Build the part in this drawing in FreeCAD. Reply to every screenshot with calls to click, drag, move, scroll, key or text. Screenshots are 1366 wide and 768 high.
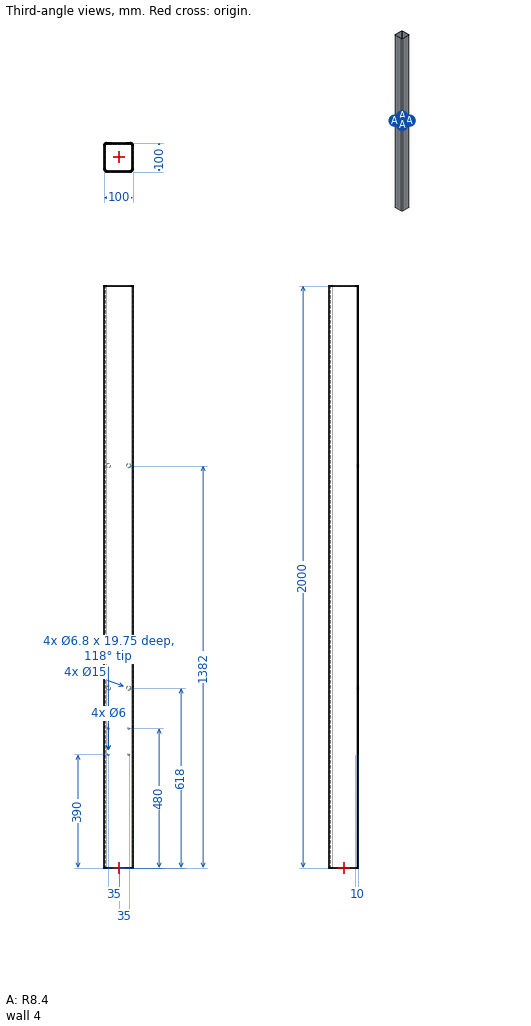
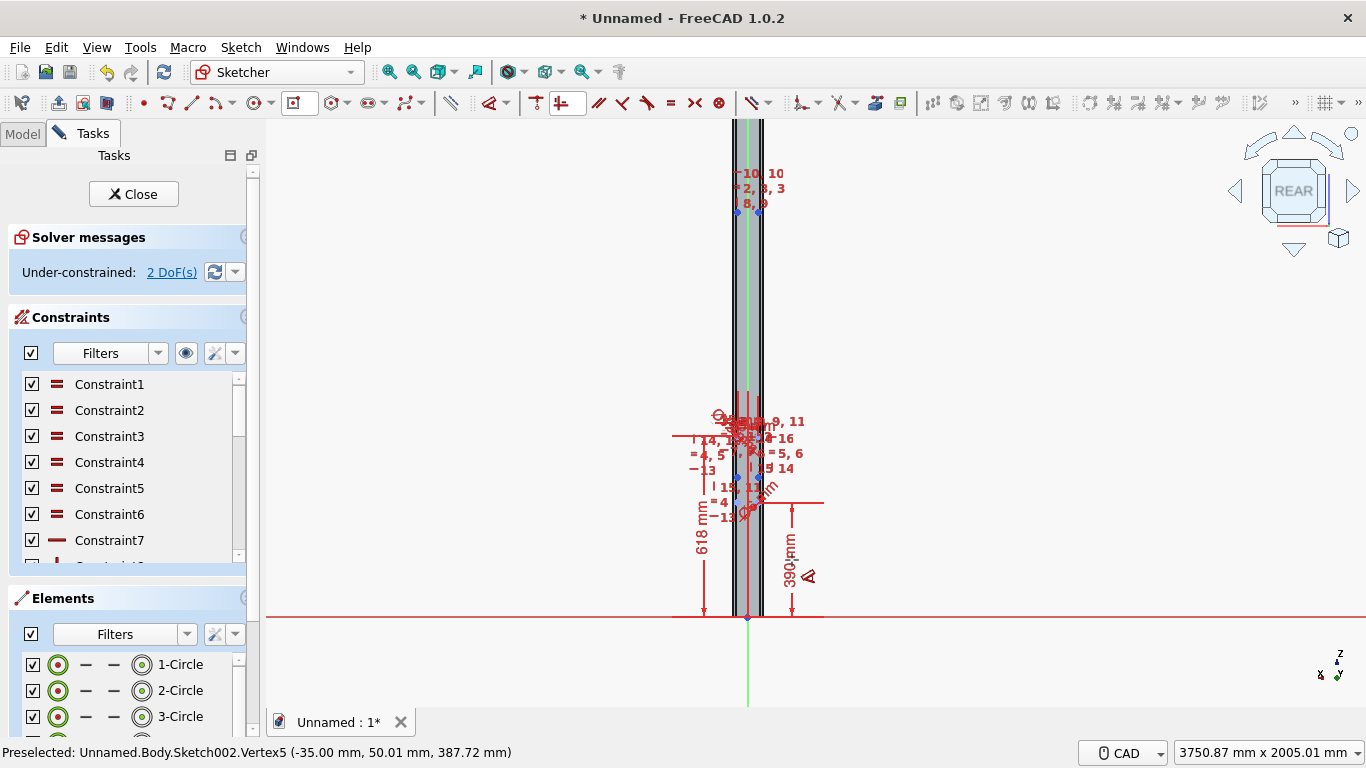
click(738, 477)
click(704, 547)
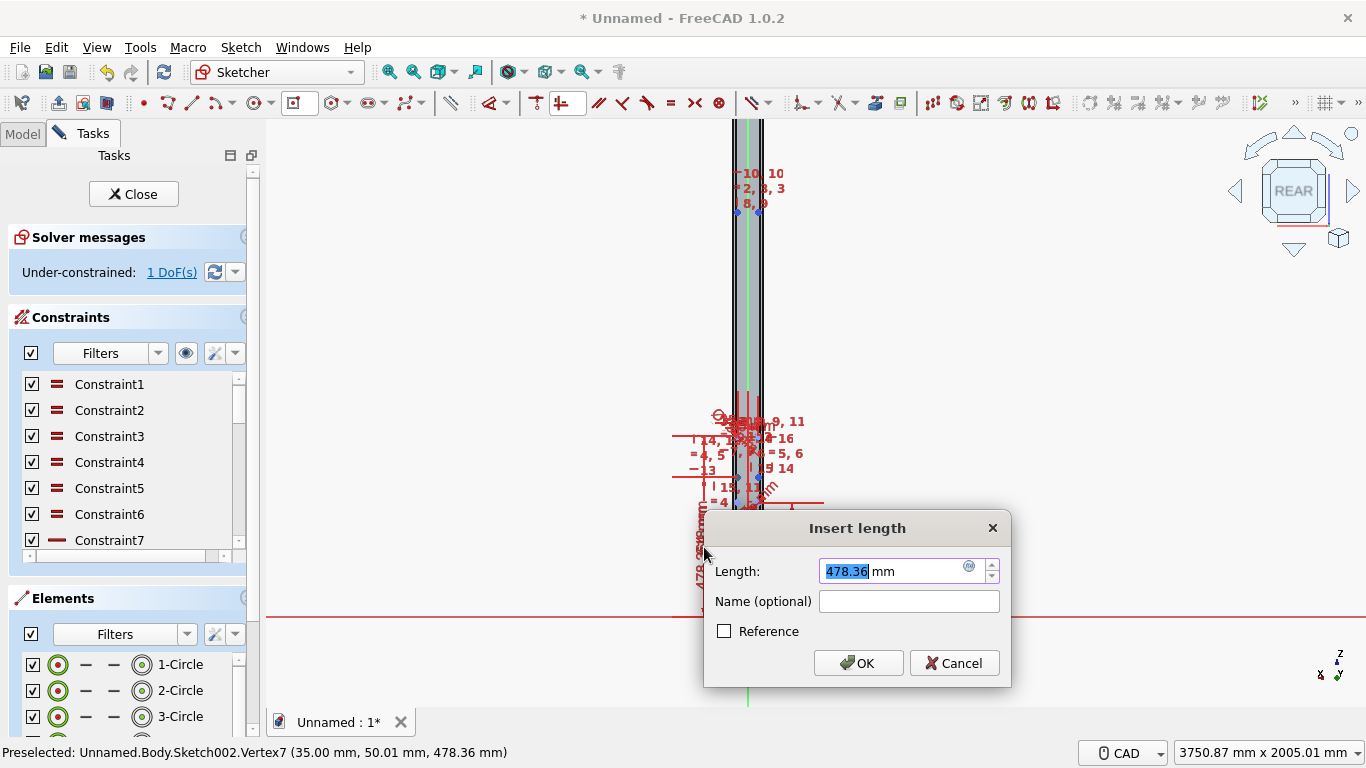
text(480)
key(Return)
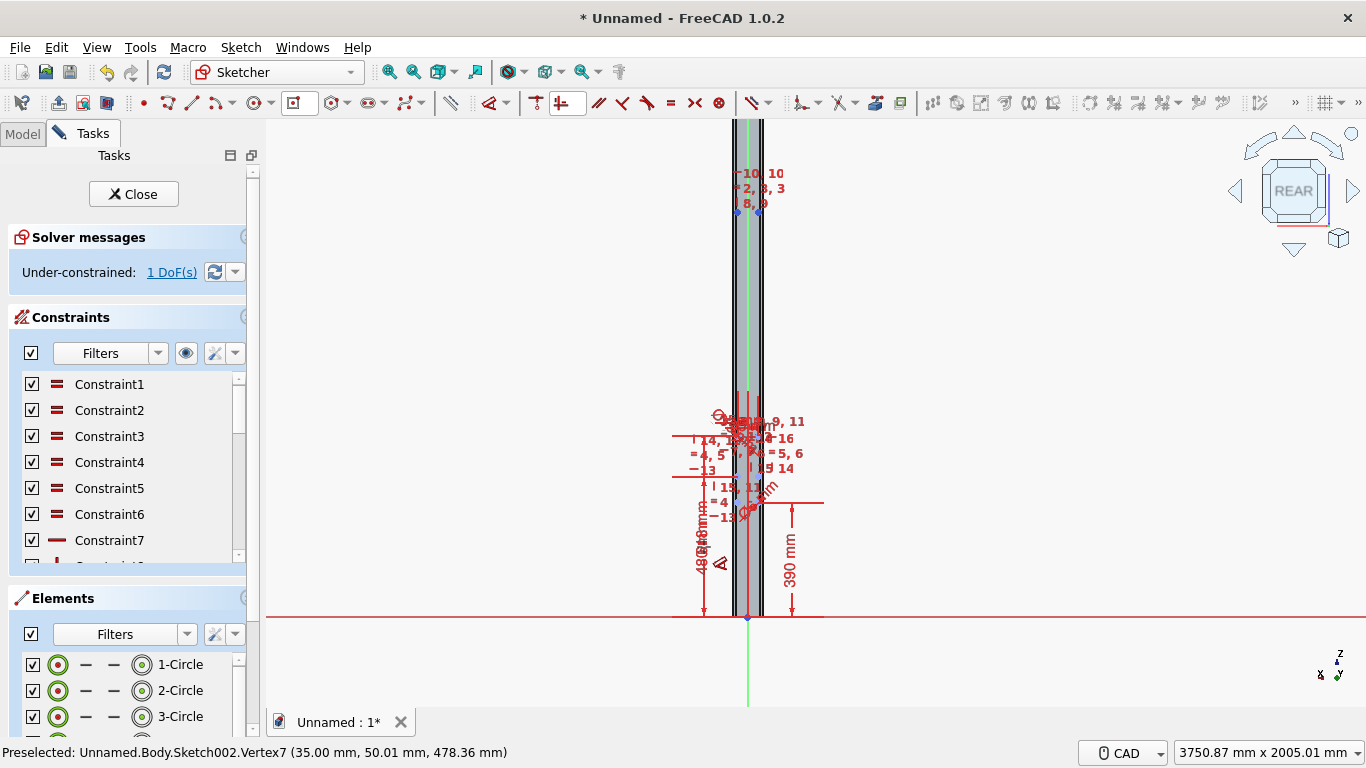
click(738, 212)
click(704, 322)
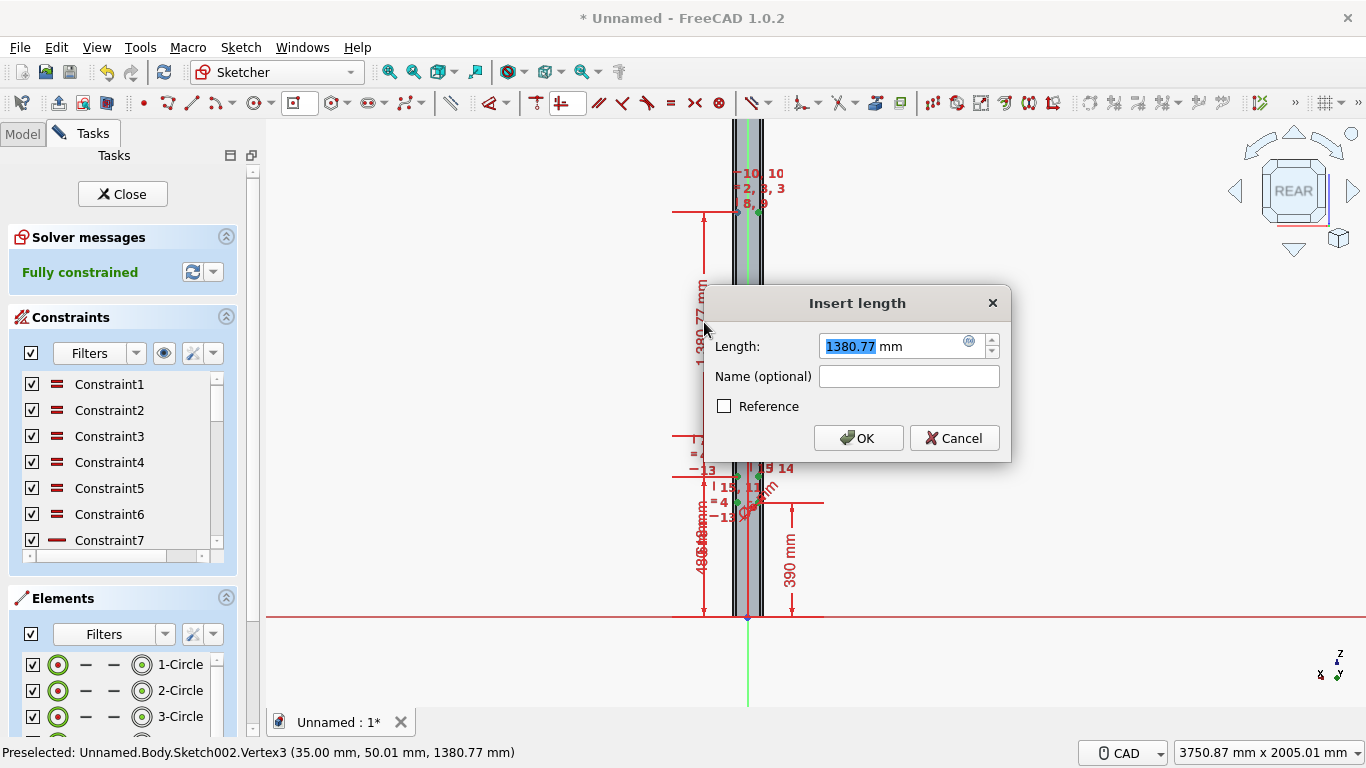
text(1382)
key(Return)
key(Escape)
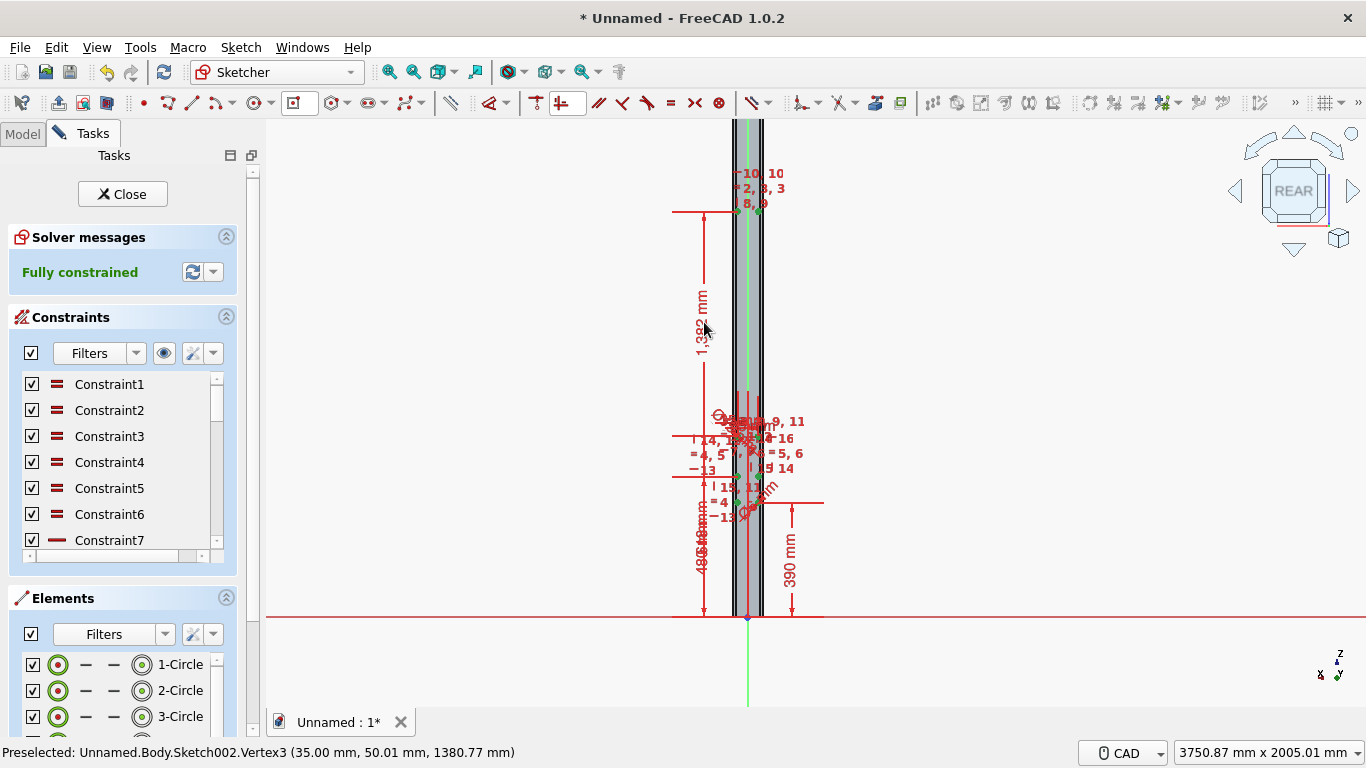
click(123, 194)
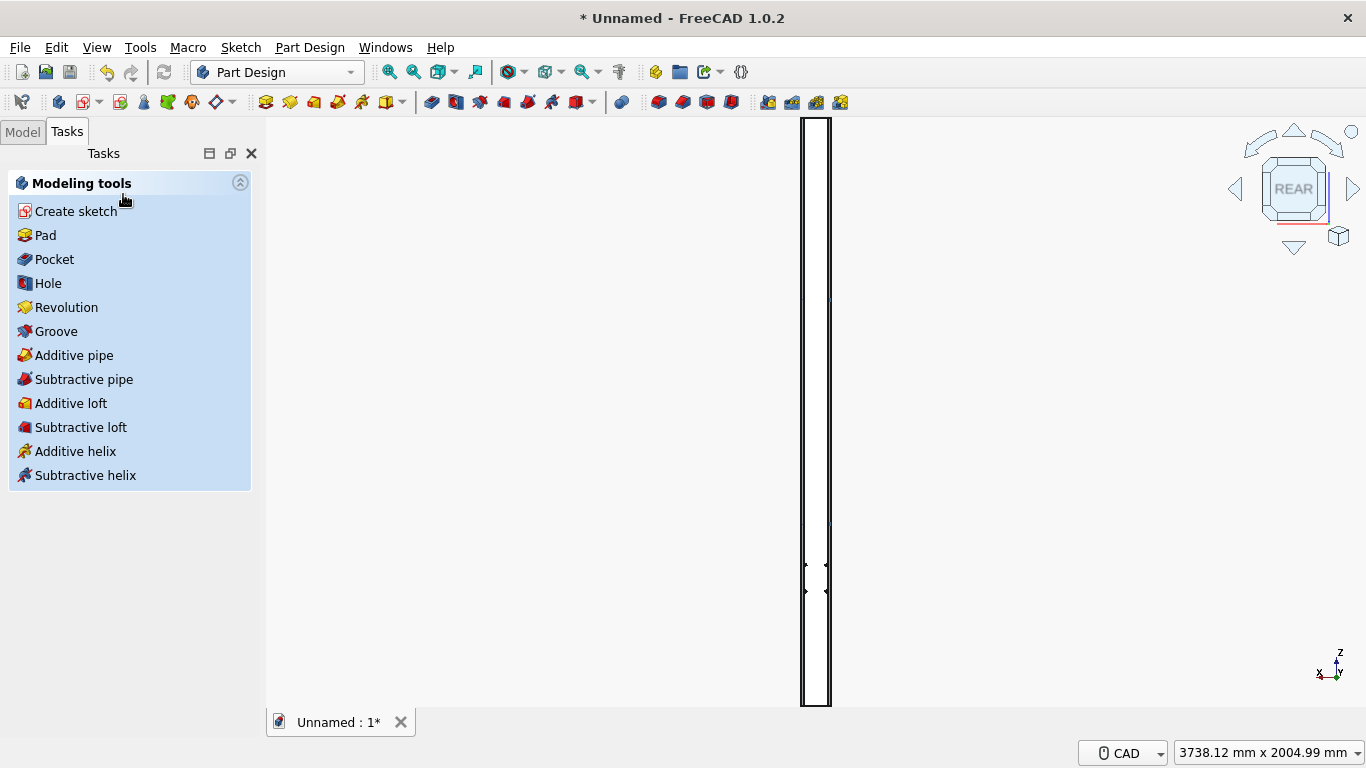
click(432, 102)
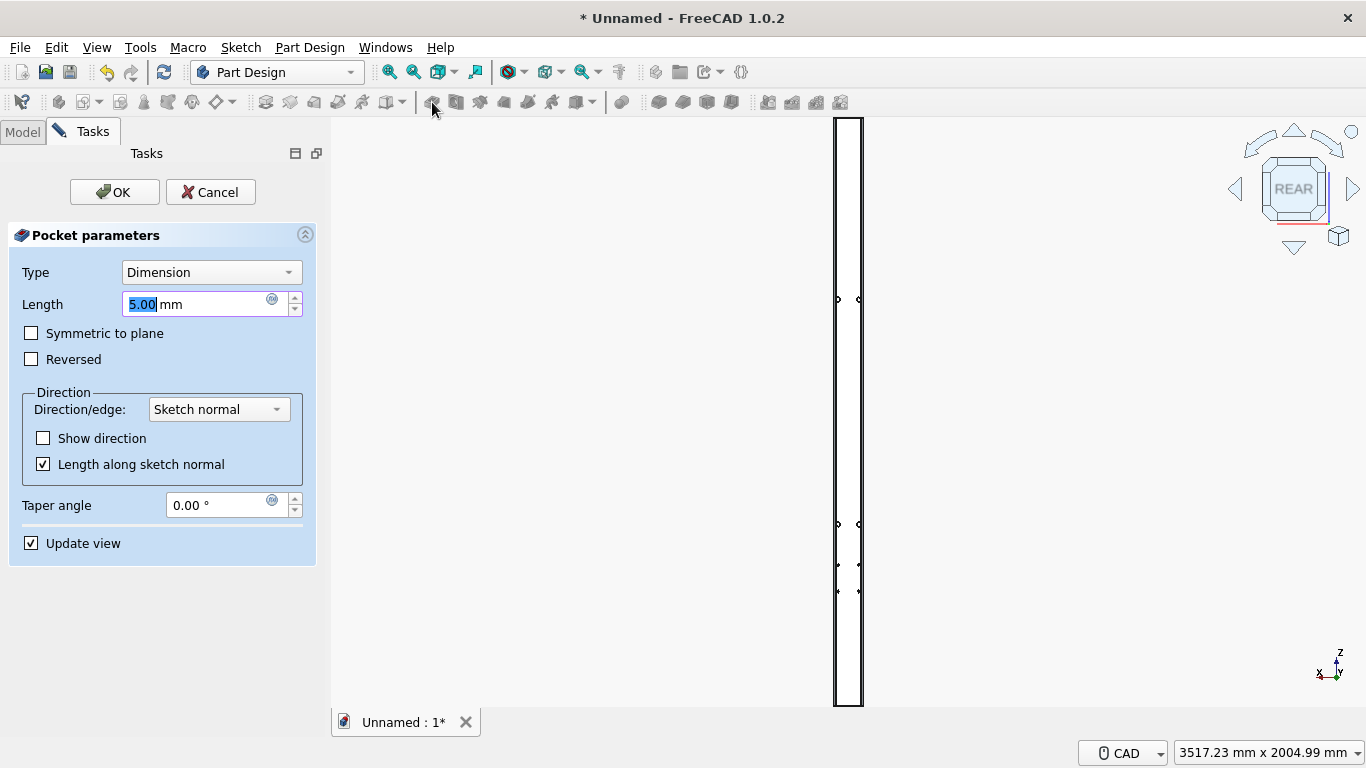
text(10)
key(Tab)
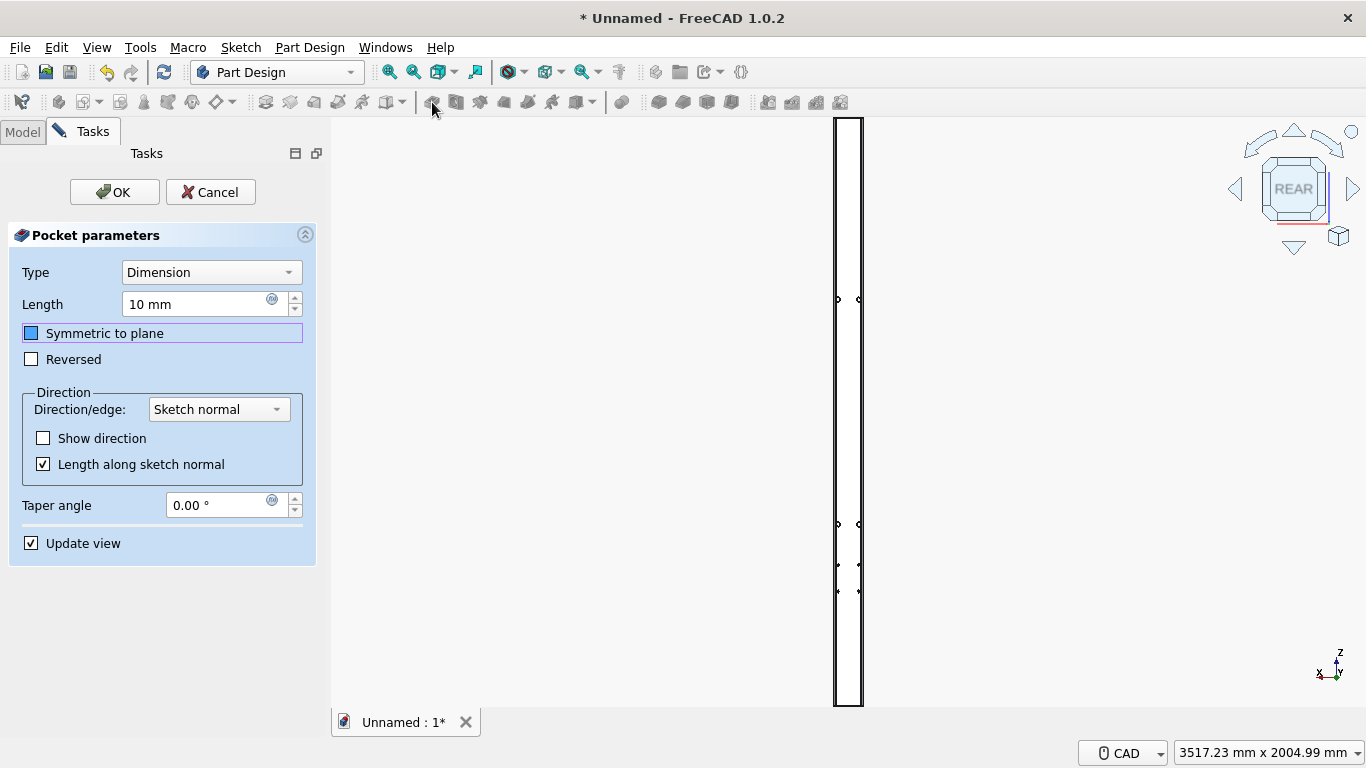
click(115, 192)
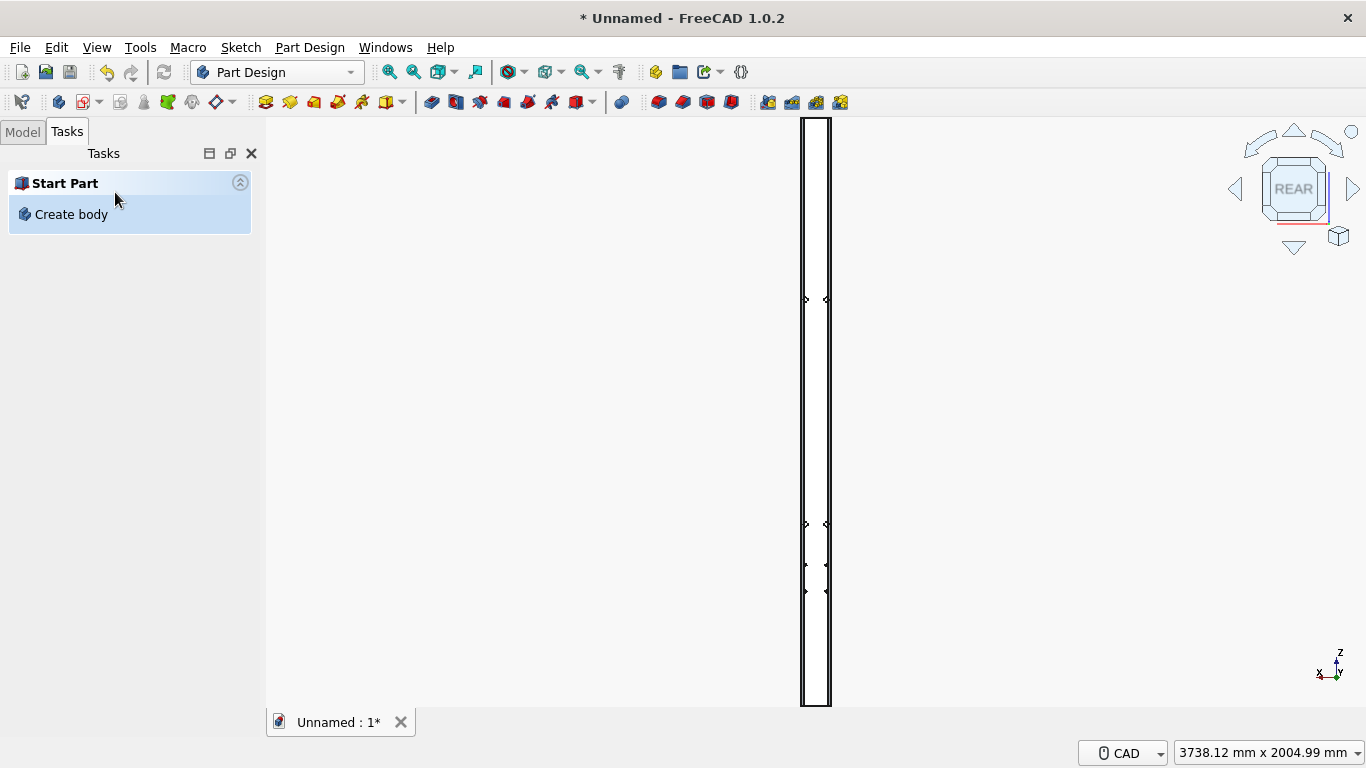
key(0)